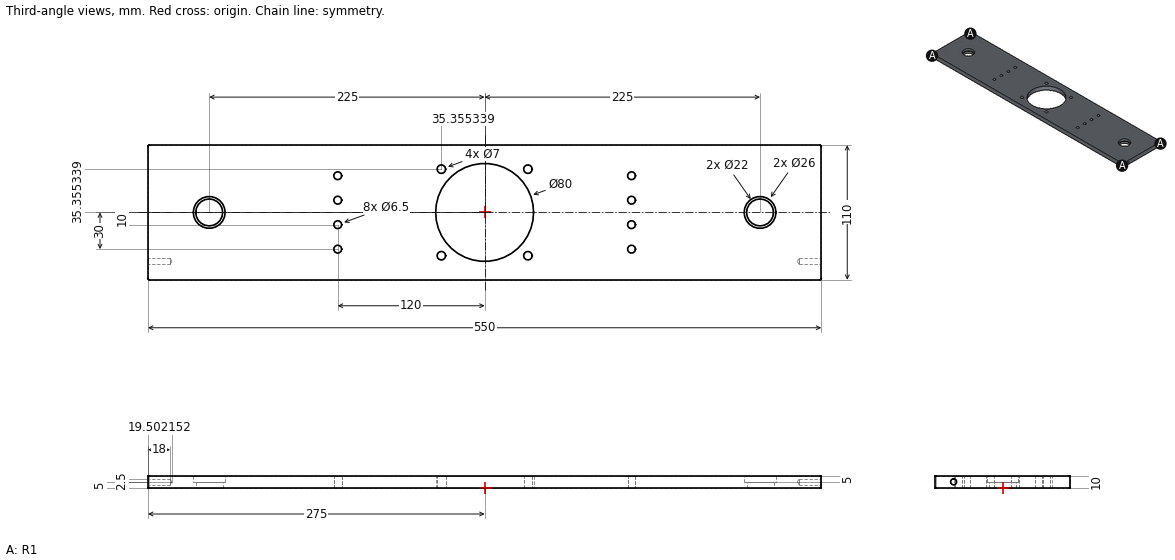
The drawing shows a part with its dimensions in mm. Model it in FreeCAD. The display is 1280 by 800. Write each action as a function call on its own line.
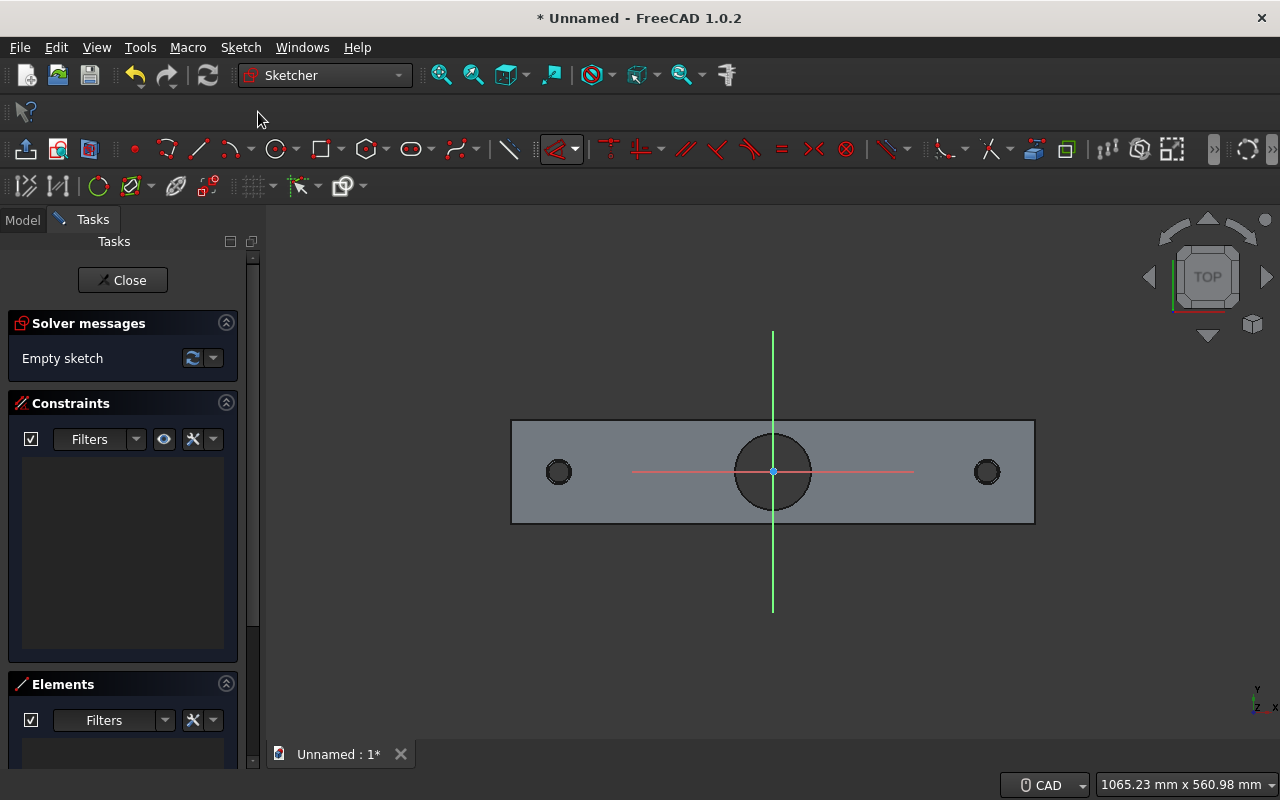
scroll(790, 472, up, 8)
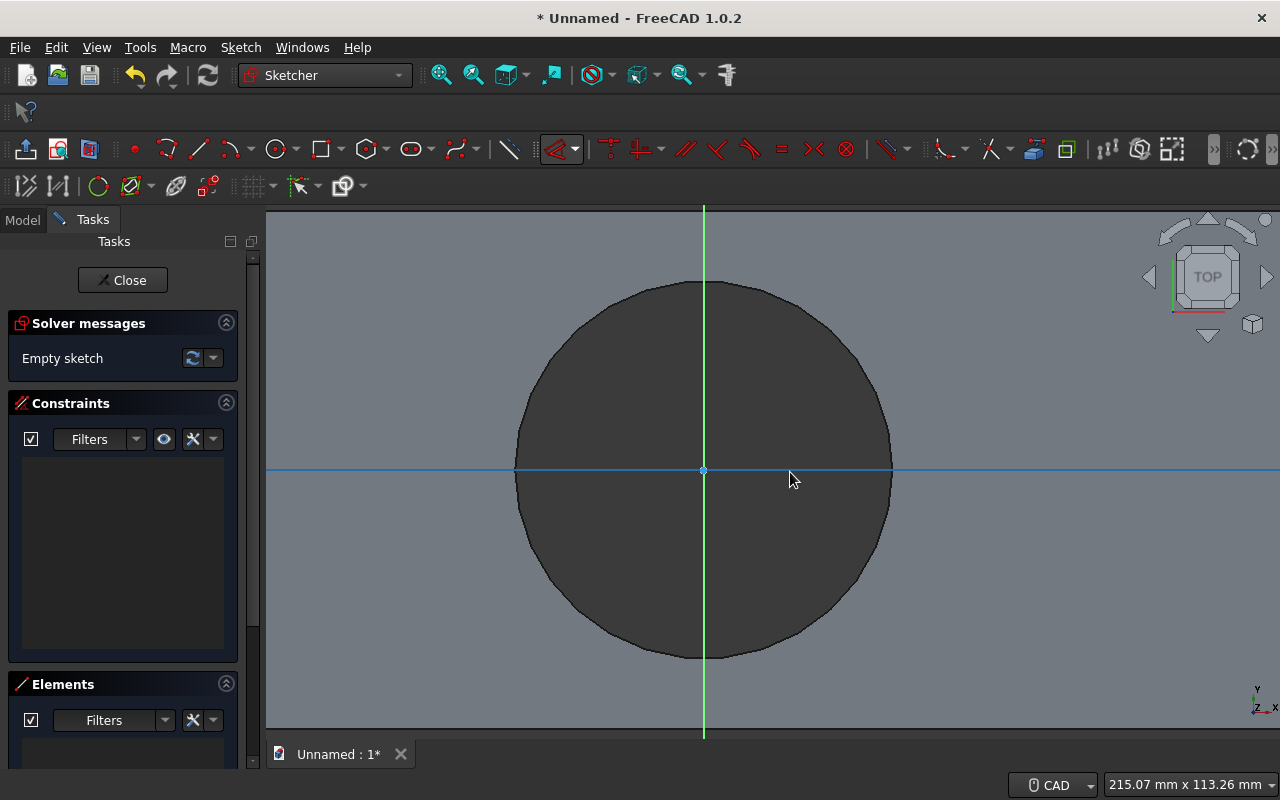
key(g)
key(c)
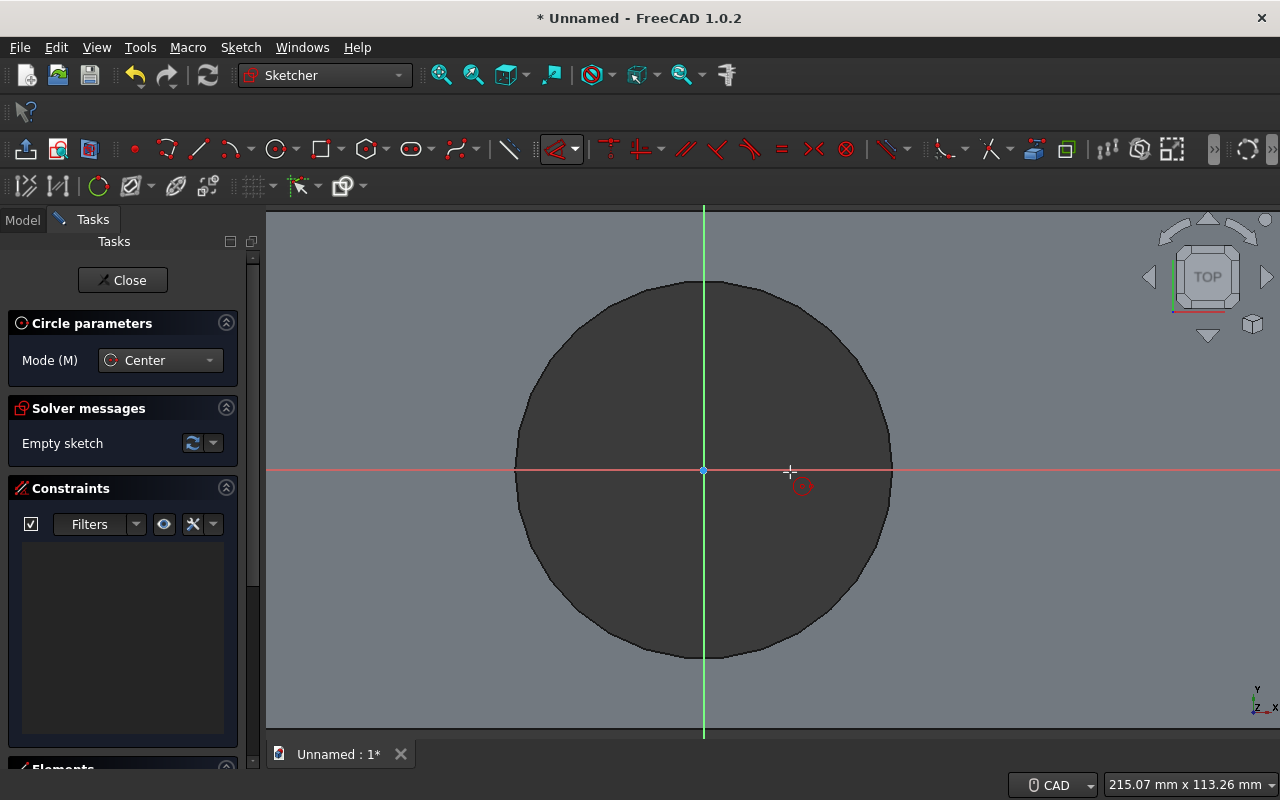
scroll(537, 303, up, 2)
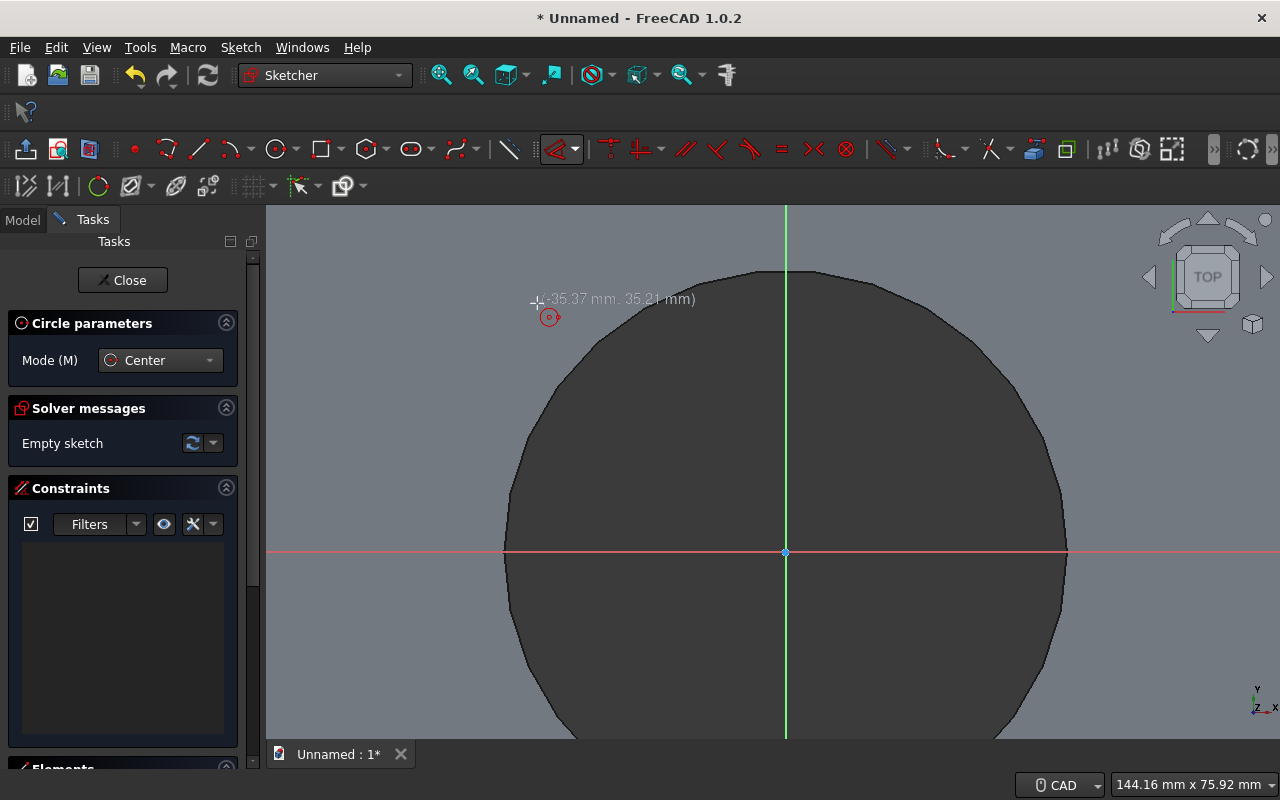
click(537, 303)
move(554, 286)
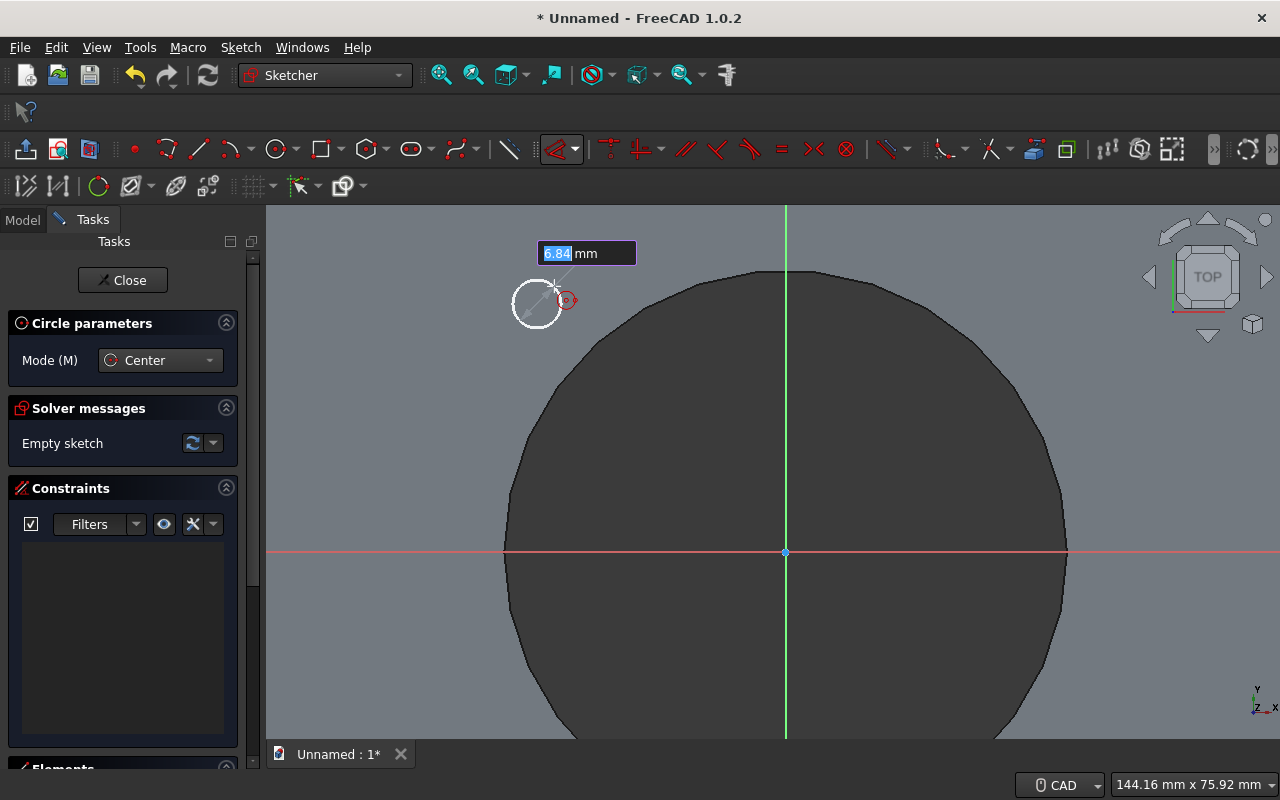
text(7)
key(Return)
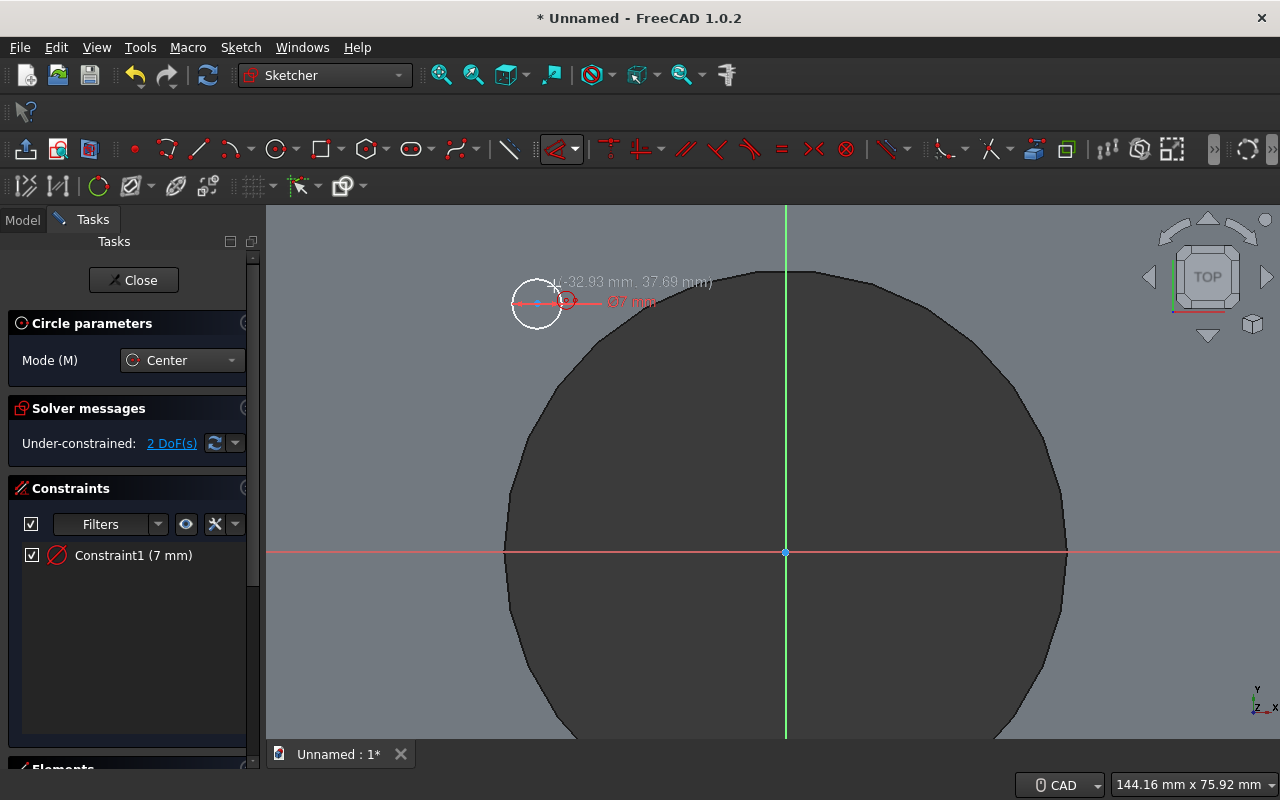
click(1034, 303)
move(1052, 286)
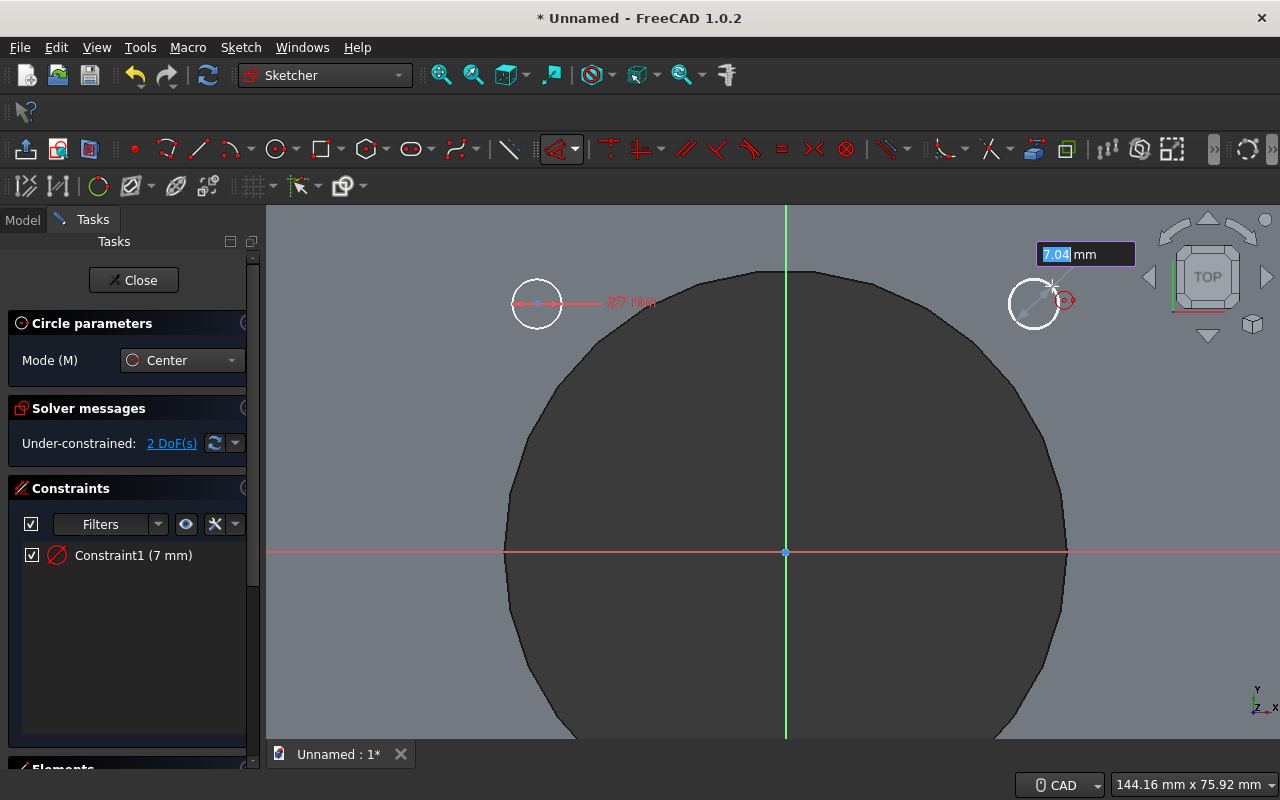
text(7)
key(Return)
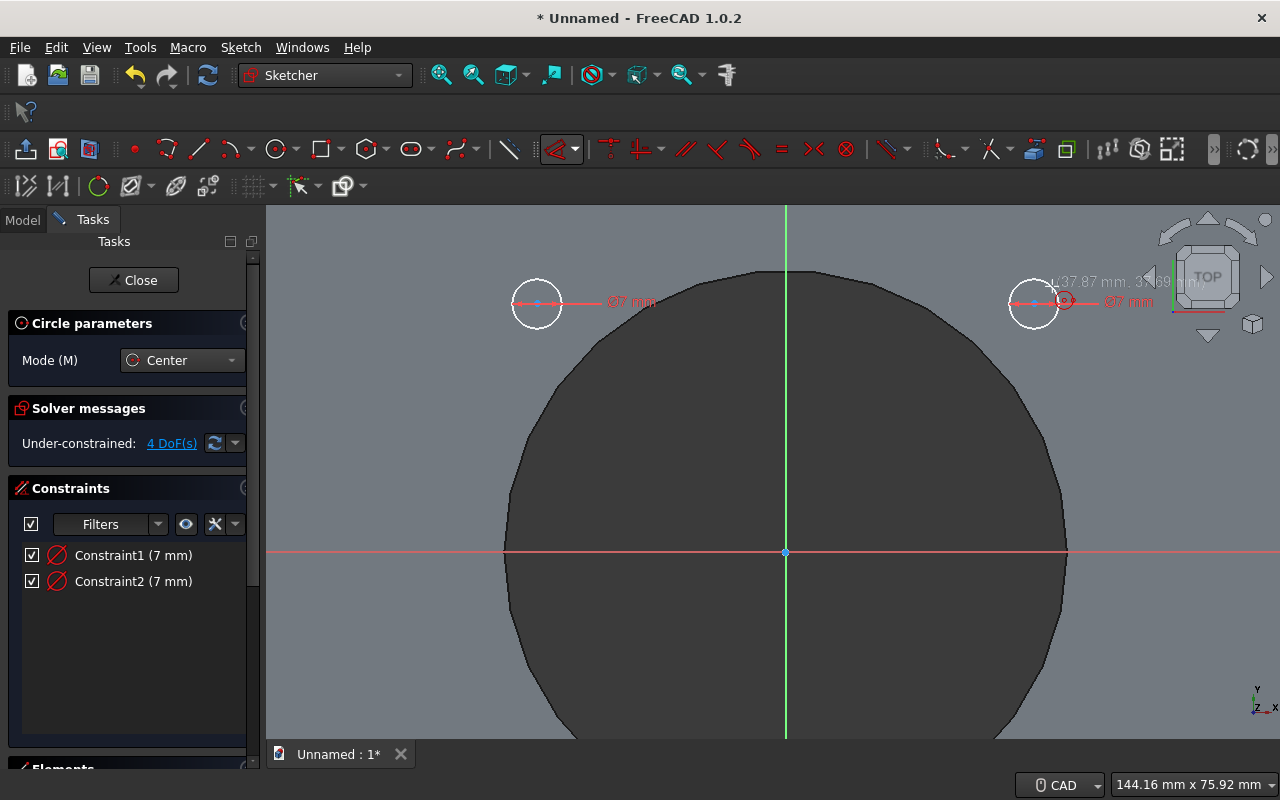
scroll(540, 309, down, 2)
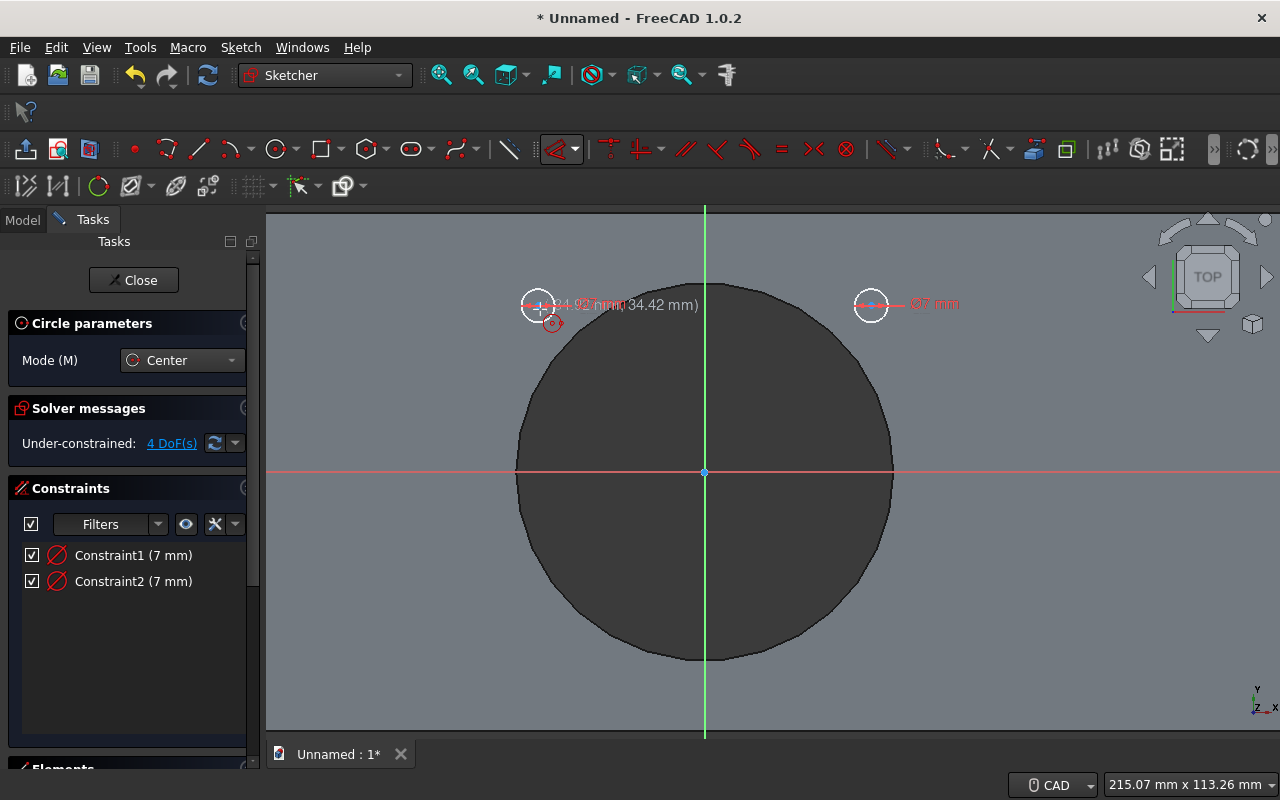
scroll(871, 639, up, 2)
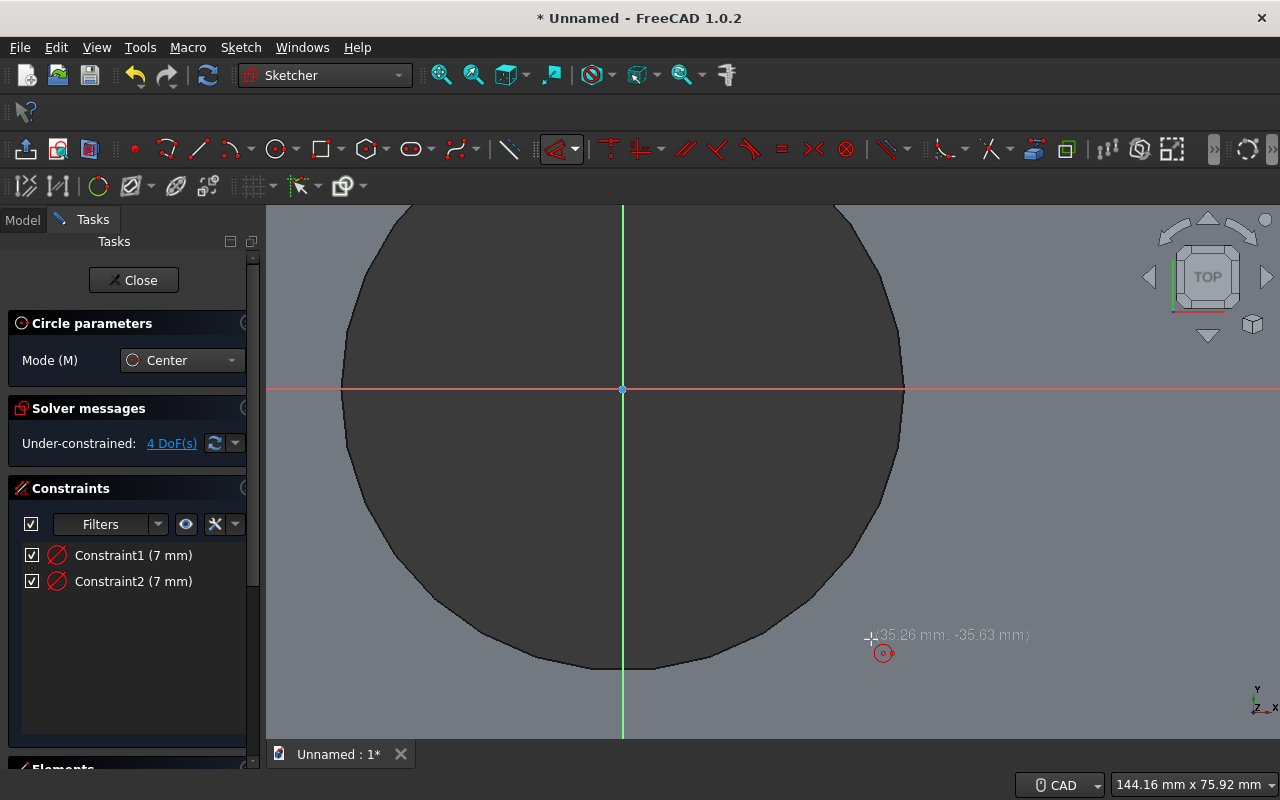
click(871, 638)
move(889, 621)